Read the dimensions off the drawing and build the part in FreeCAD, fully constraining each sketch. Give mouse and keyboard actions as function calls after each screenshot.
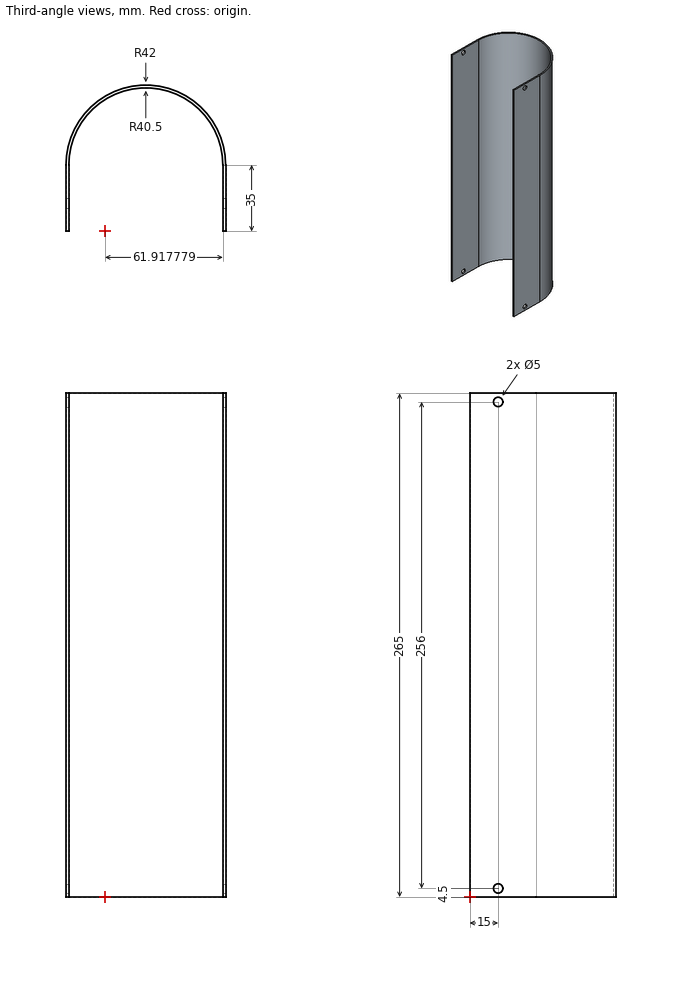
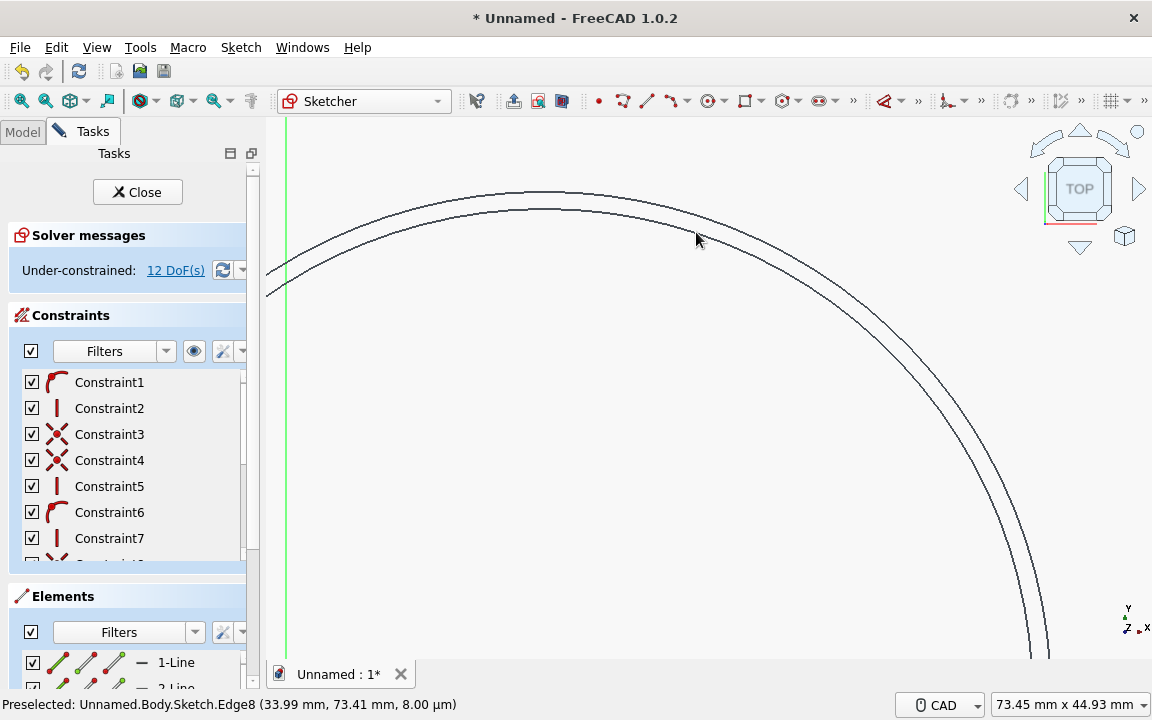
scroll(696, 233, down, 5)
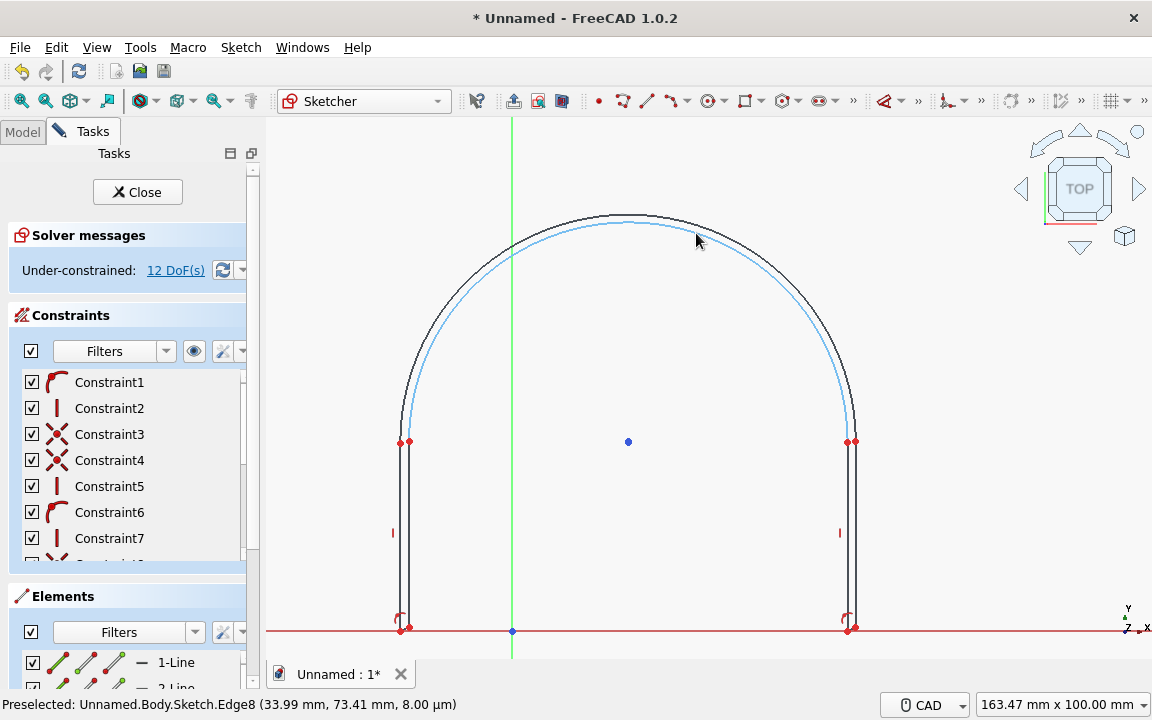
scroll(824, 557, up, 8)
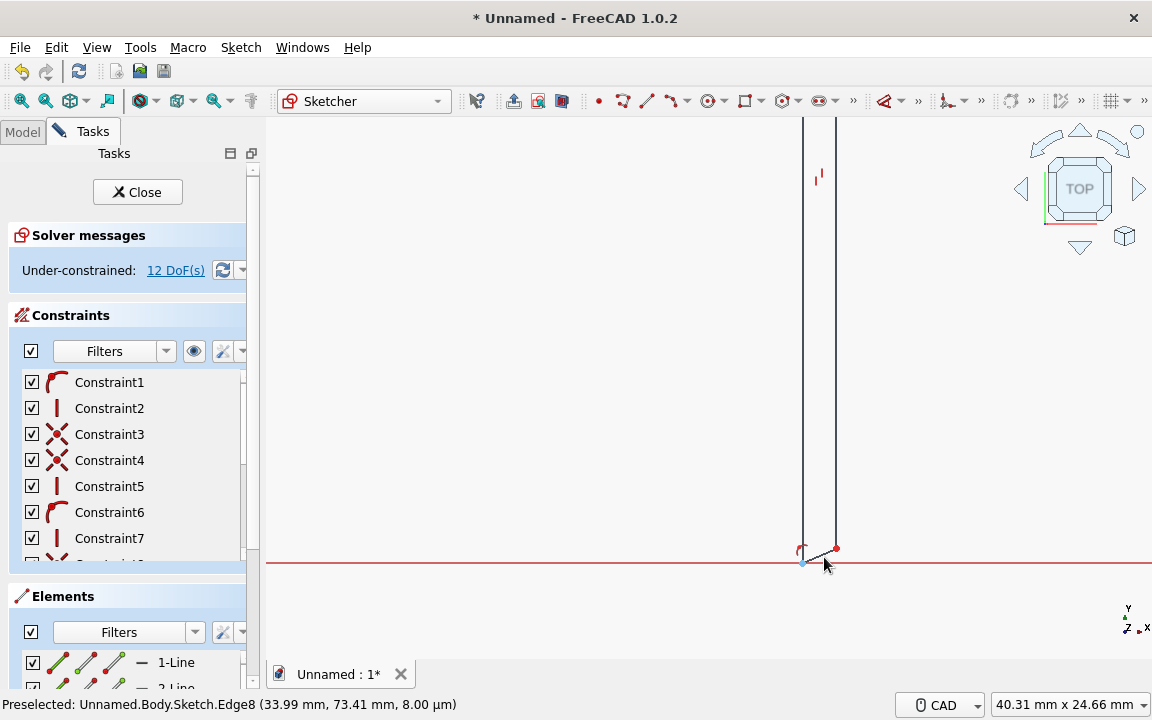
click(819, 556)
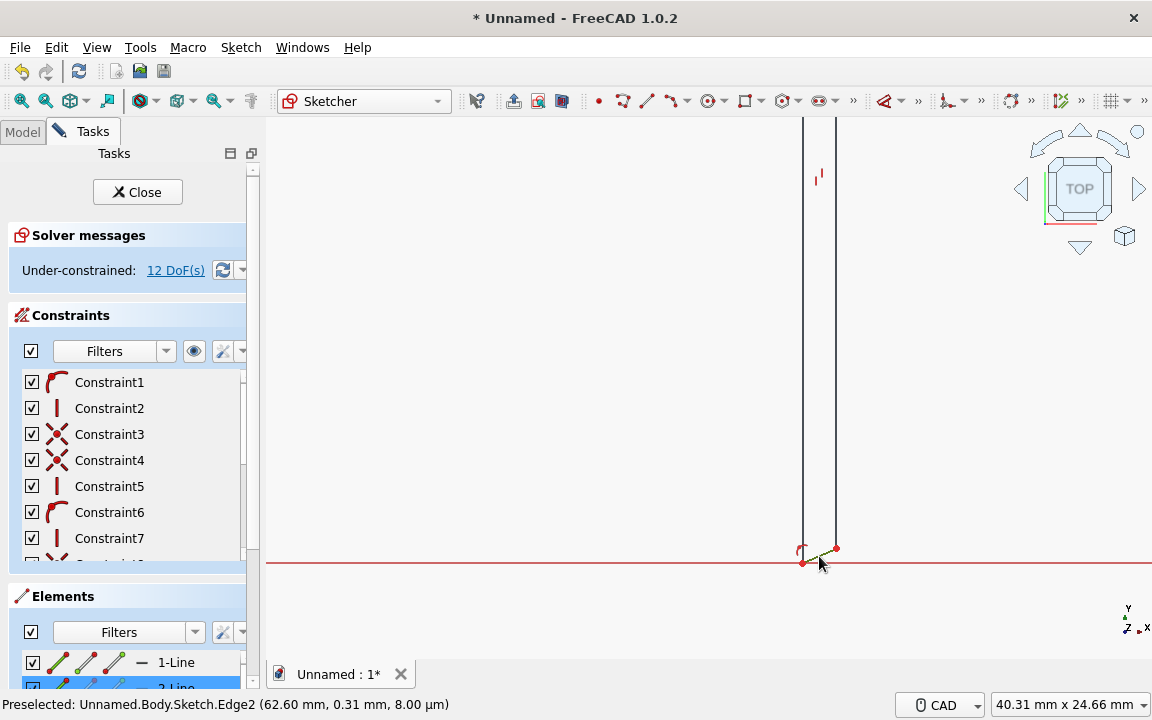
key(h)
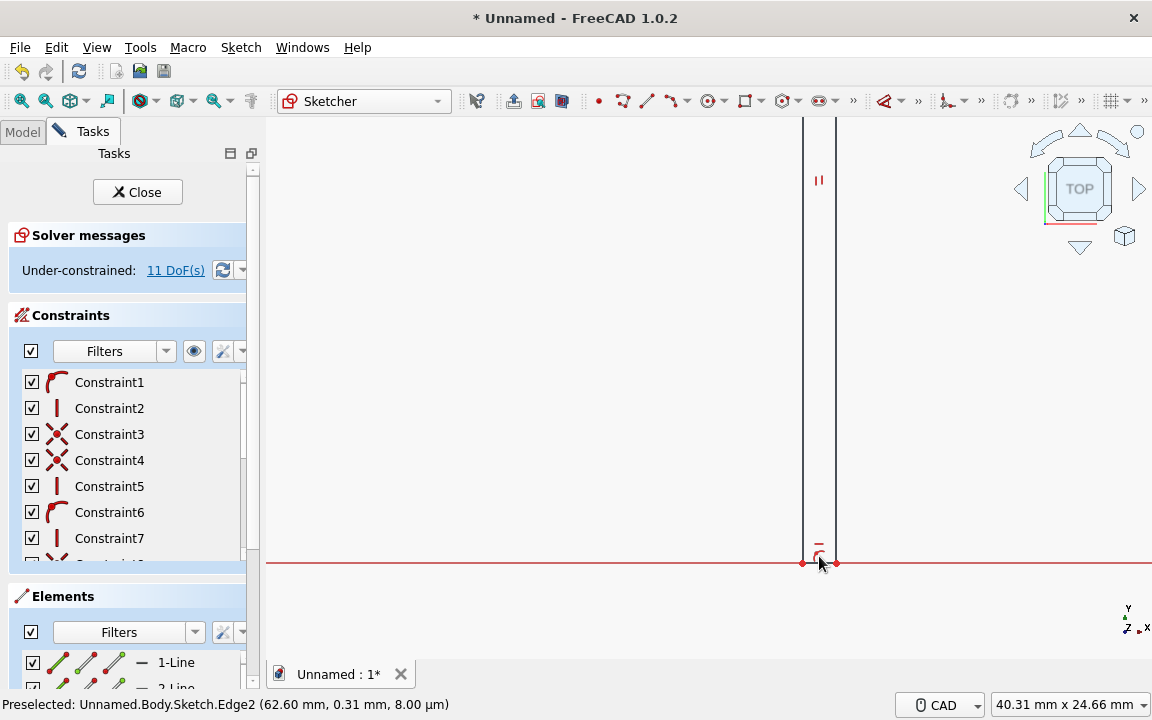
scroll(824, 558, down, 8)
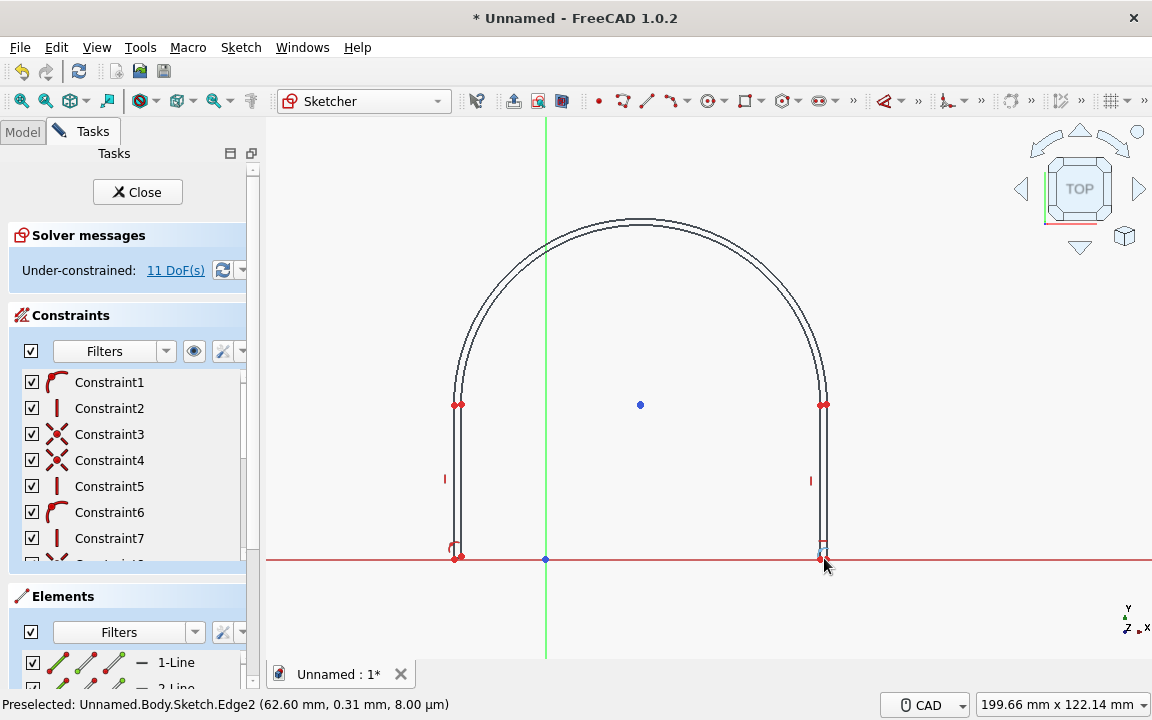
scroll(459, 558, up, 10)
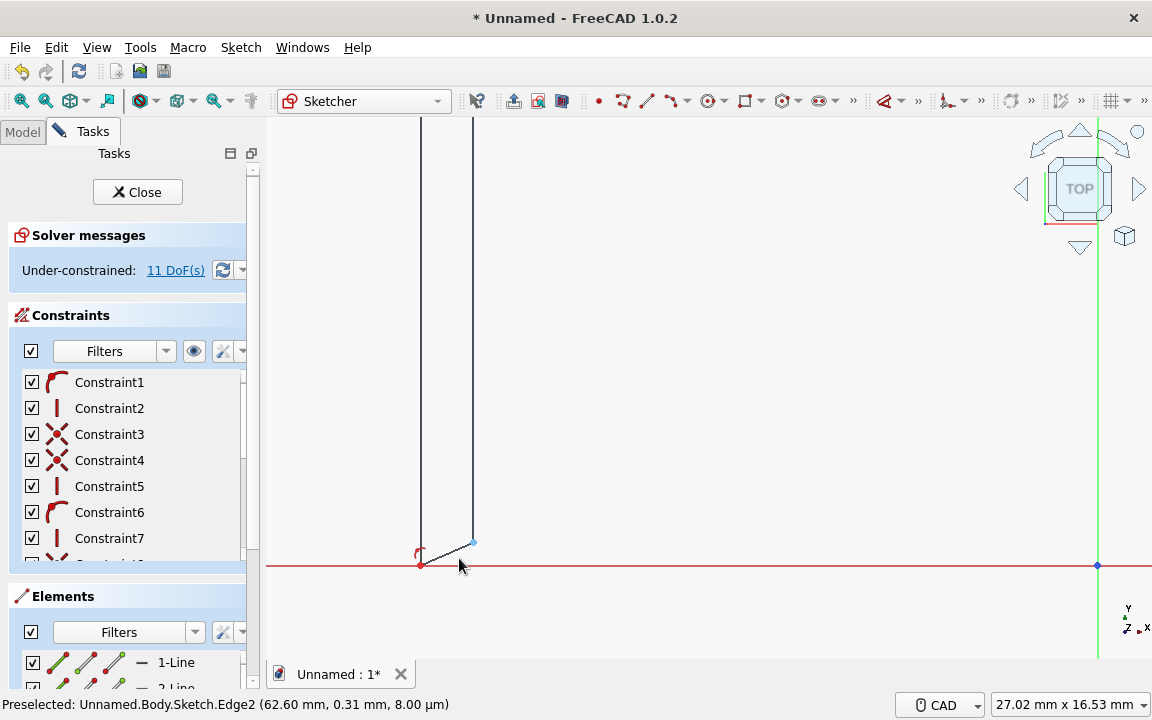
click(458, 550)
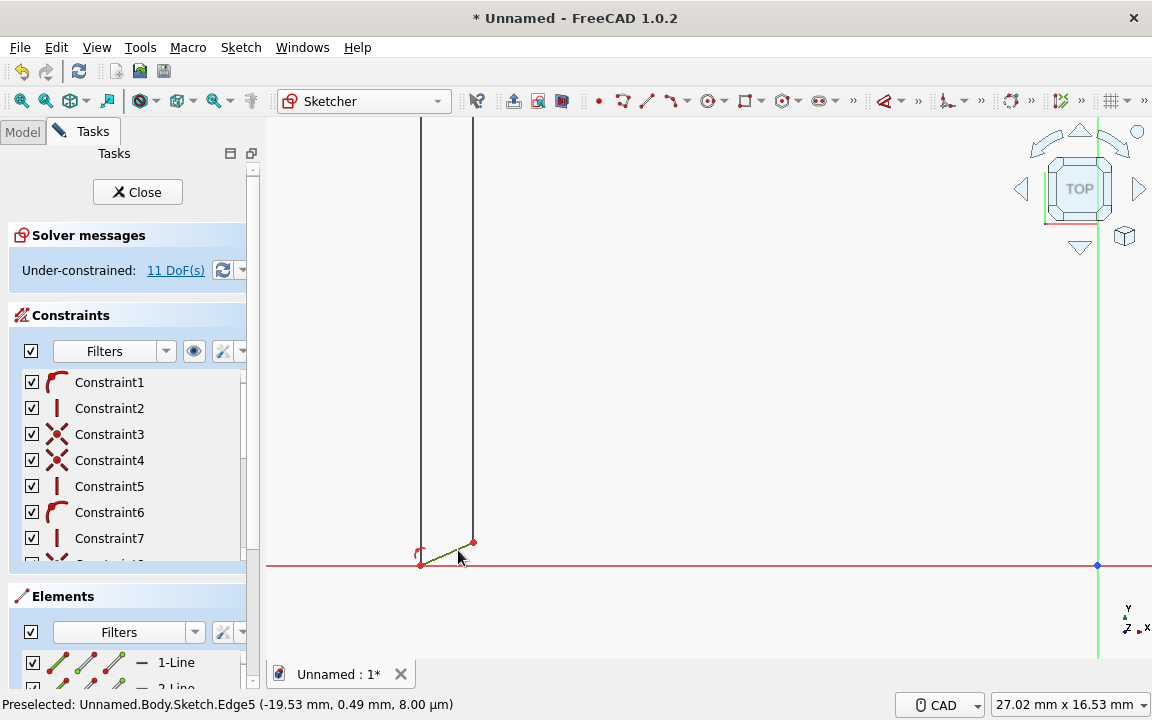
key(h)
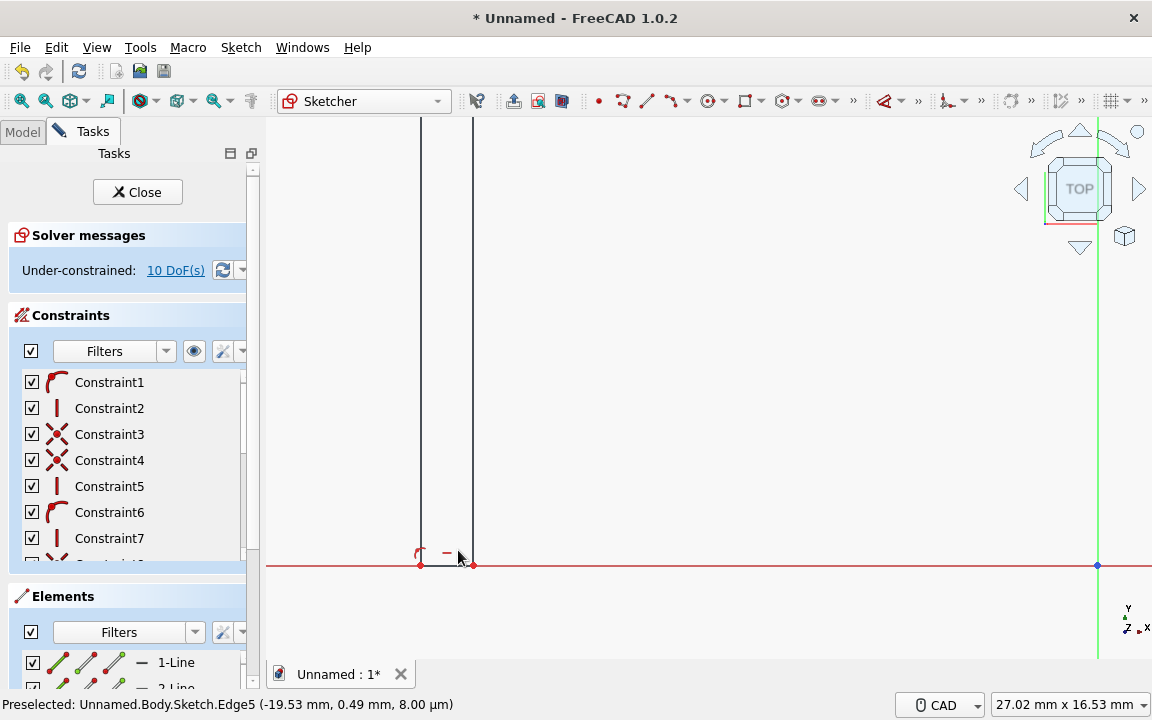
scroll(459, 558, down, 10)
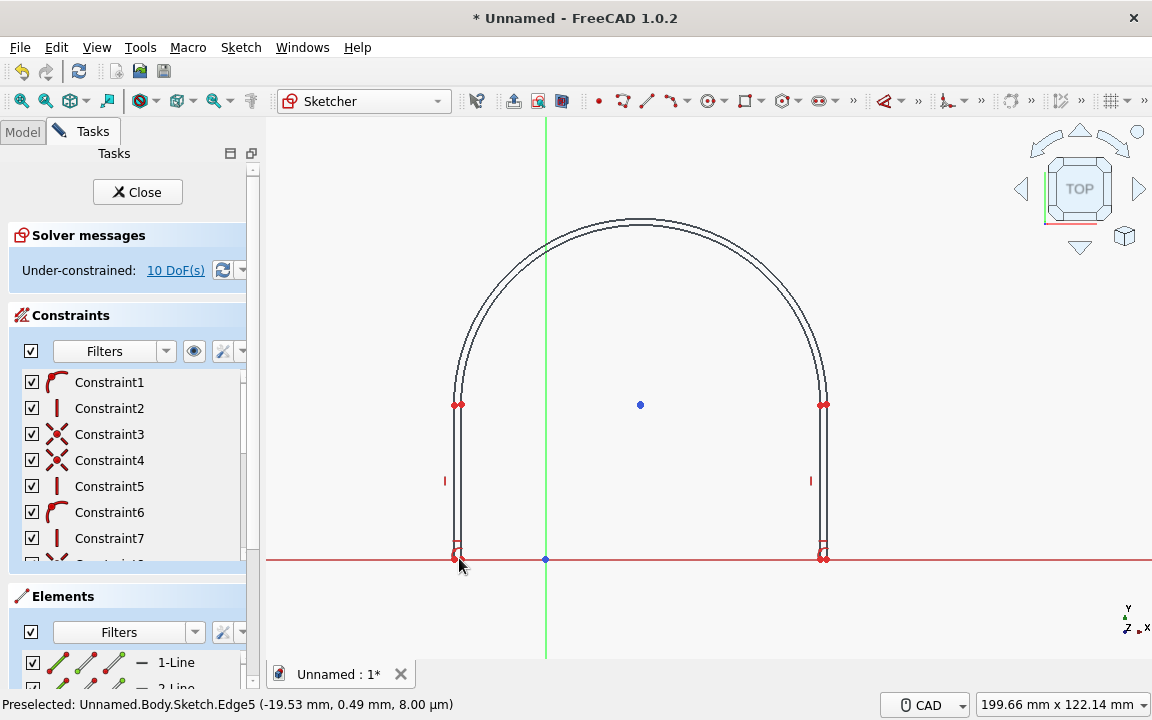
scroll(750, 254, up, 4)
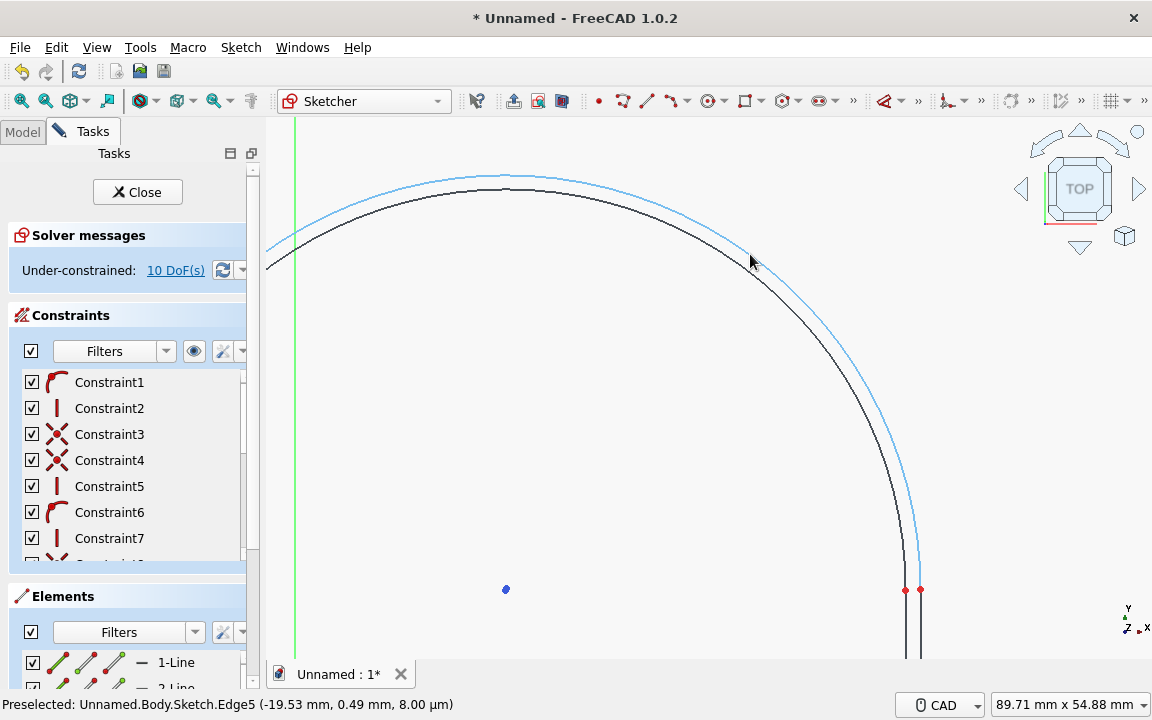
click(749, 254)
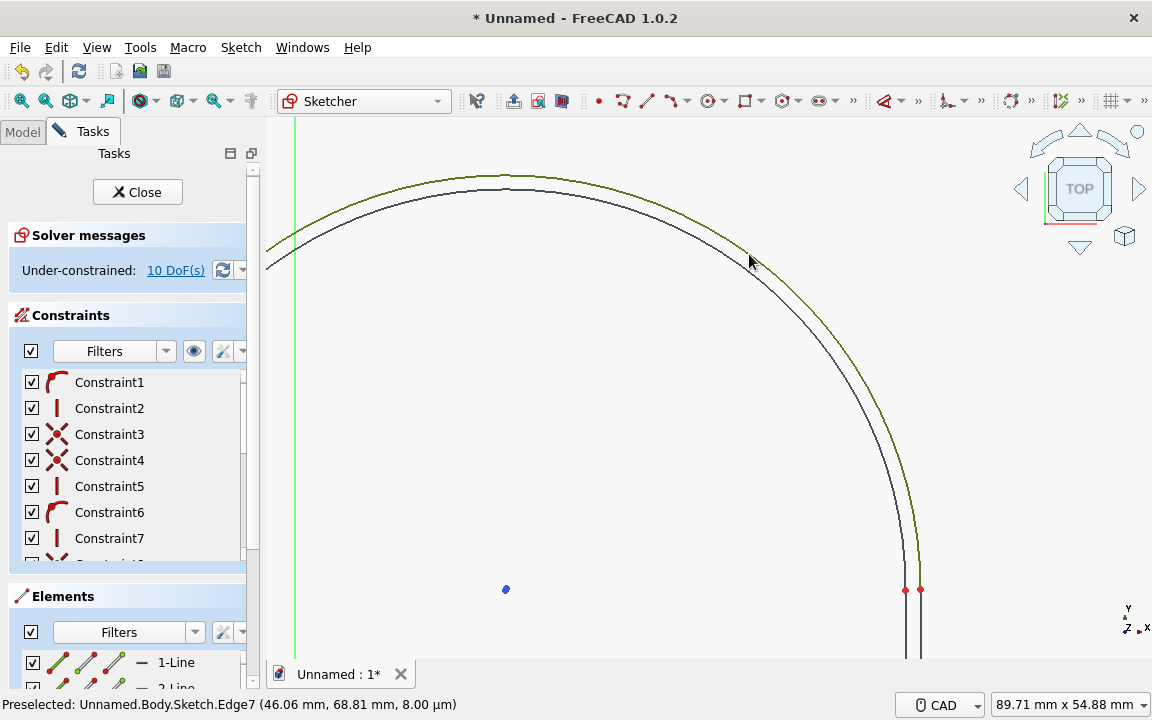
click(742, 266)